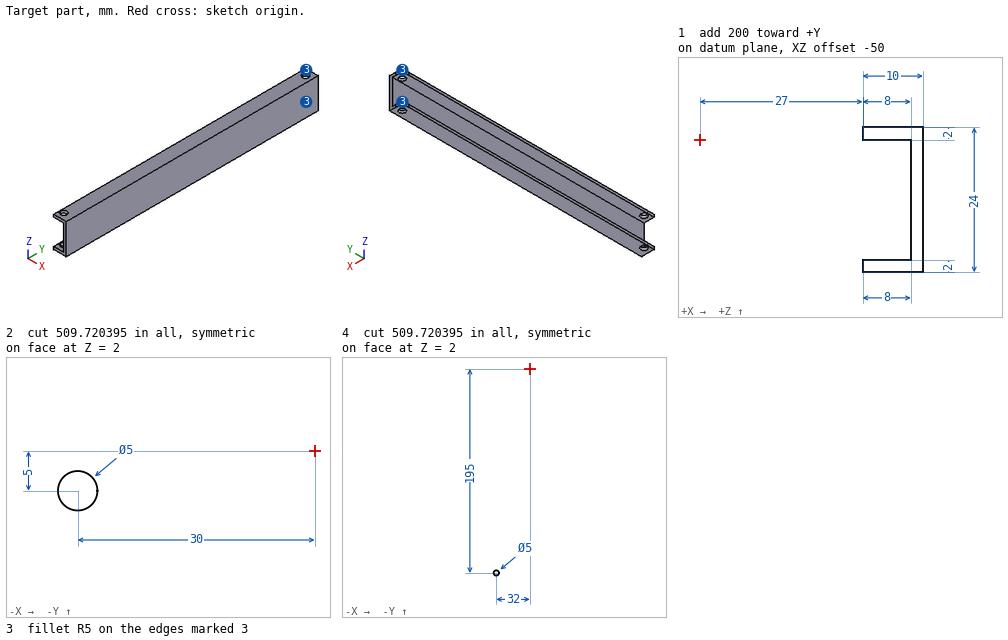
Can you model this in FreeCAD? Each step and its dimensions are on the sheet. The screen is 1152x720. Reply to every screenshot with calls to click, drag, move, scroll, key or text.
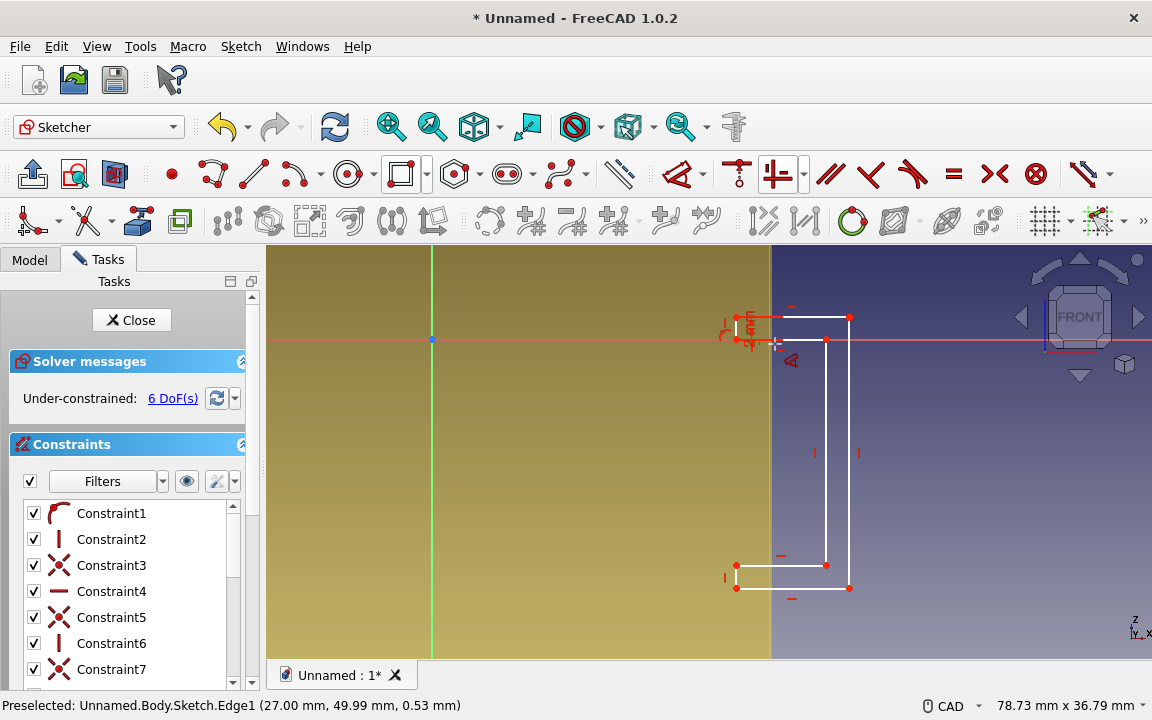
scroll(736, 582, up, 4)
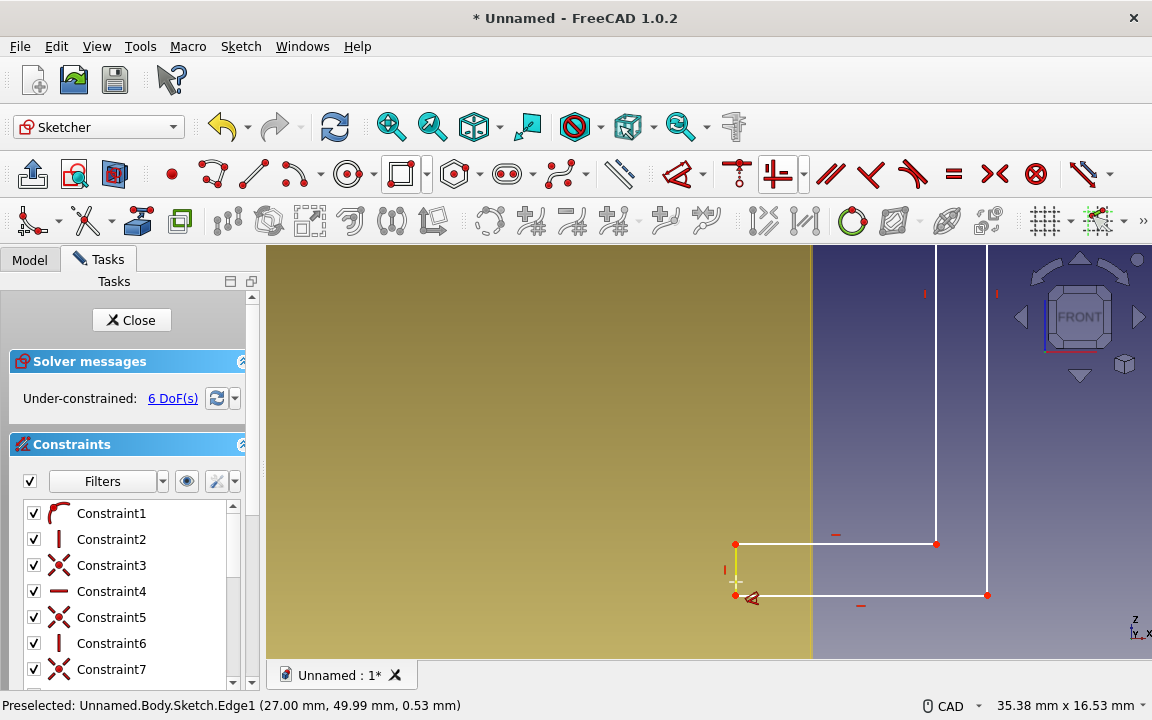
click(736, 580)
click(770, 570)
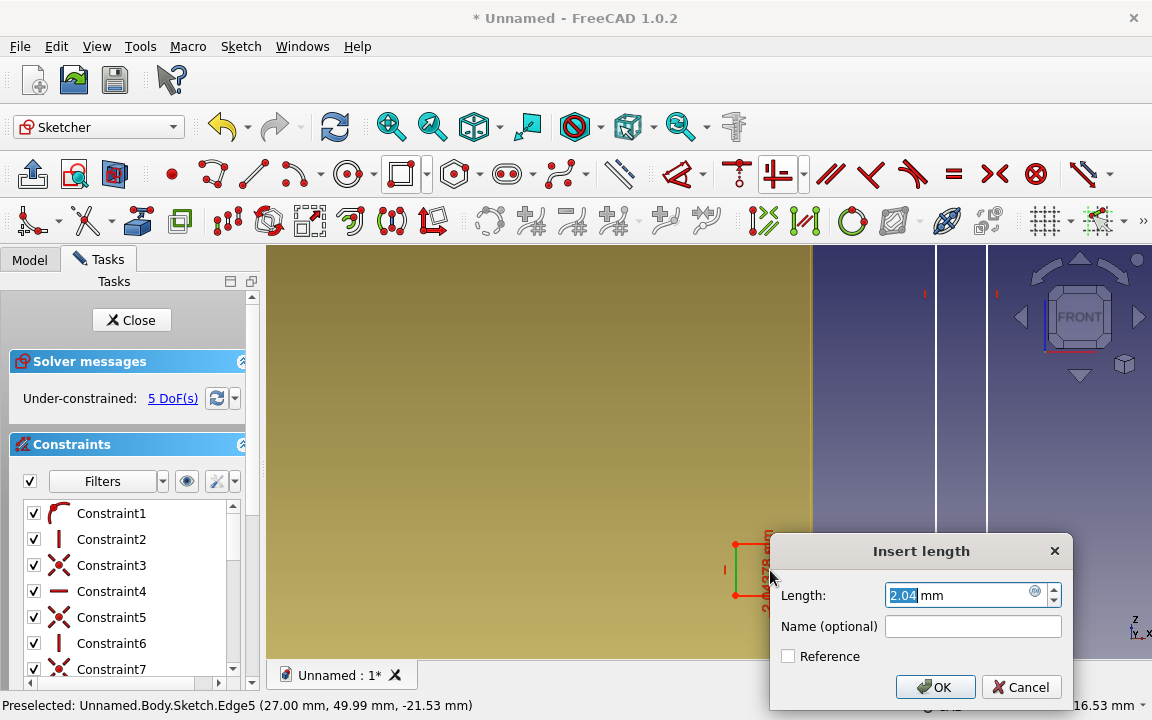
text(2)
key(Return)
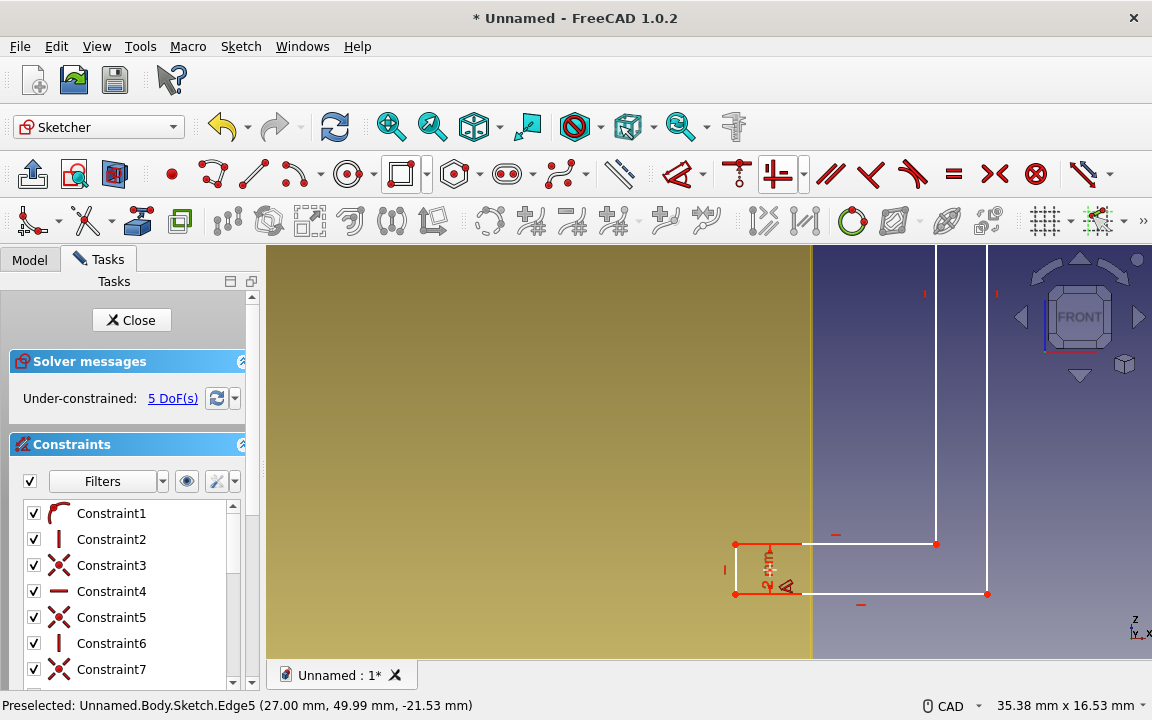
click(796, 544)
click(882, 578)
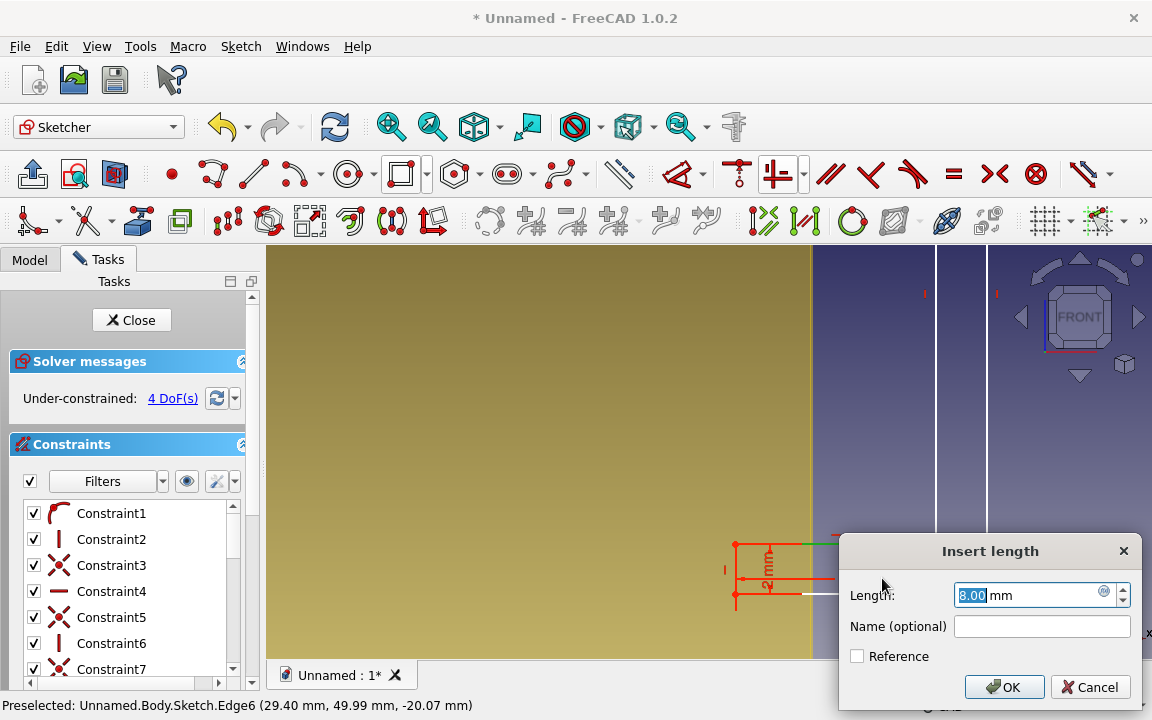
text(8)
key(Return)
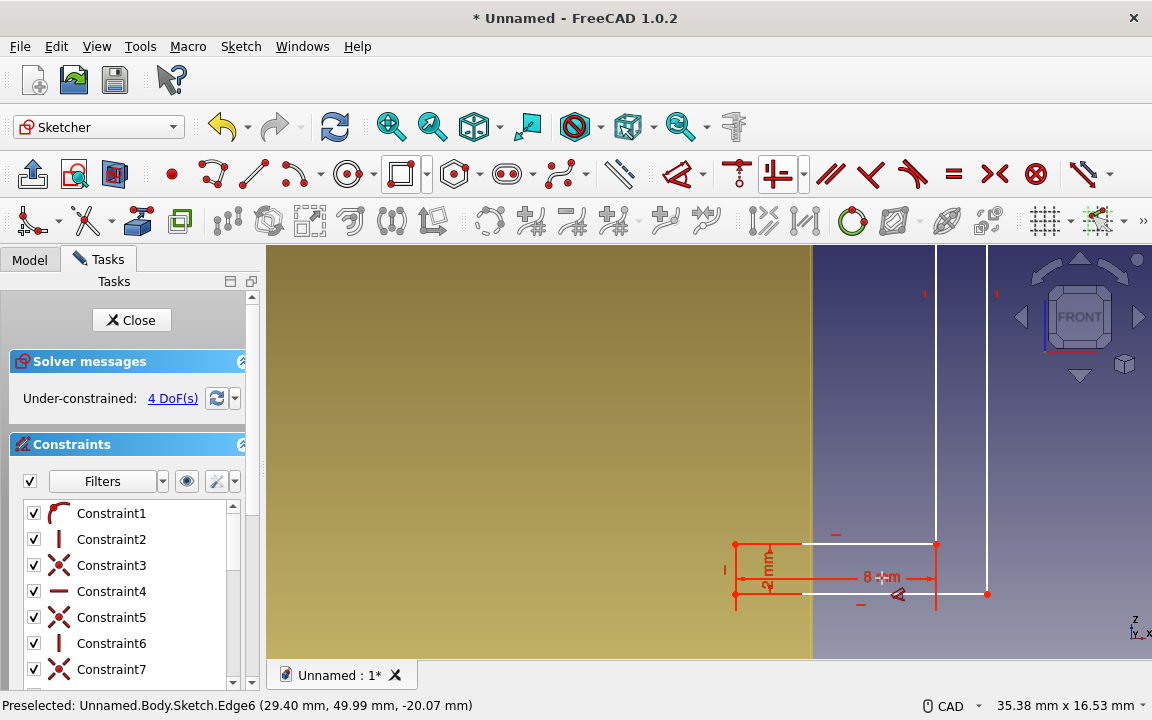
scroll(736, 582, down, 4)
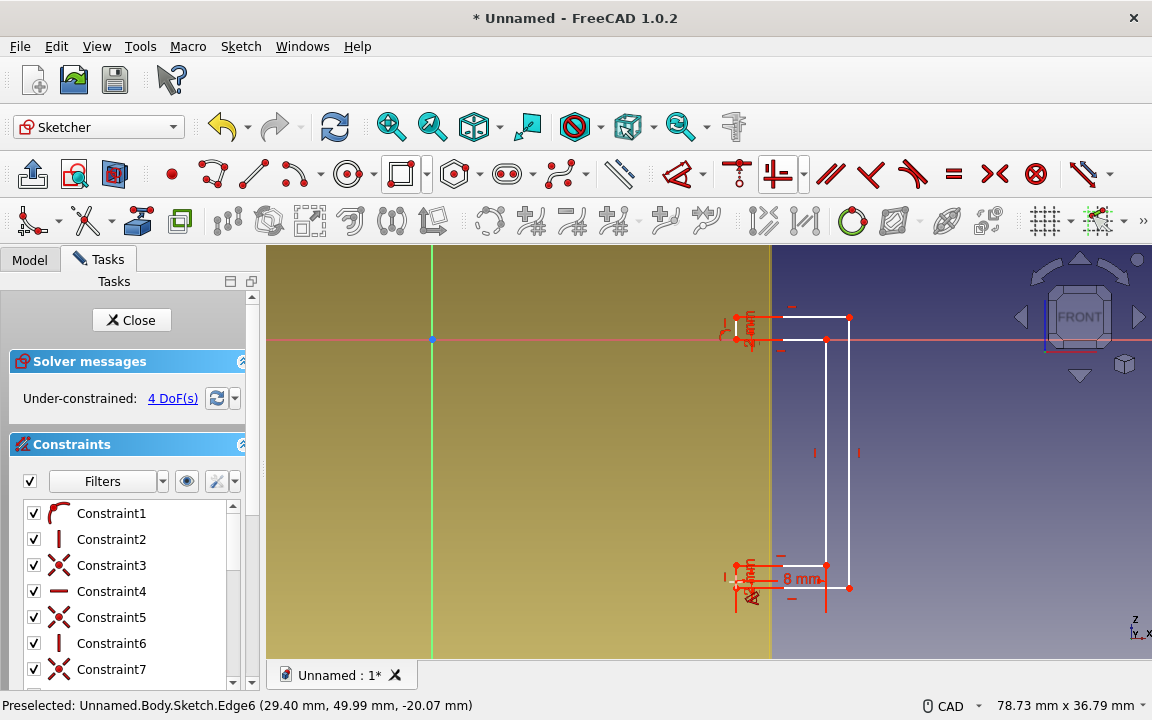
click(799, 340)
click(781, 374)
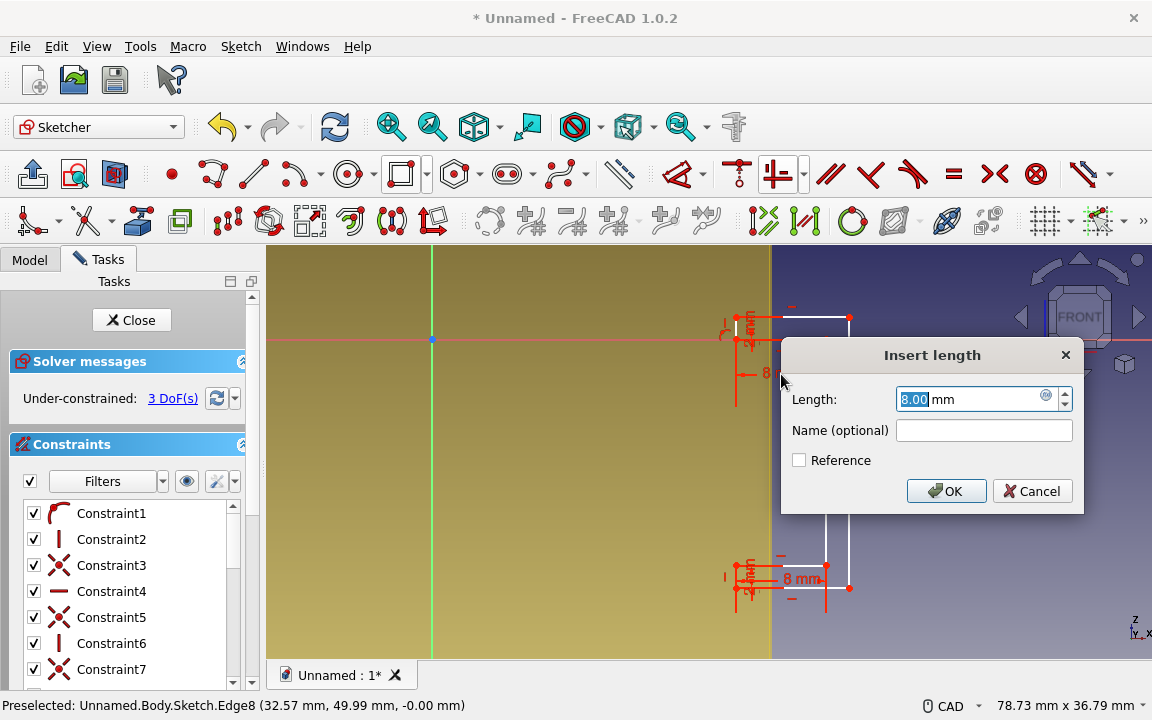
text(8)
key(Return)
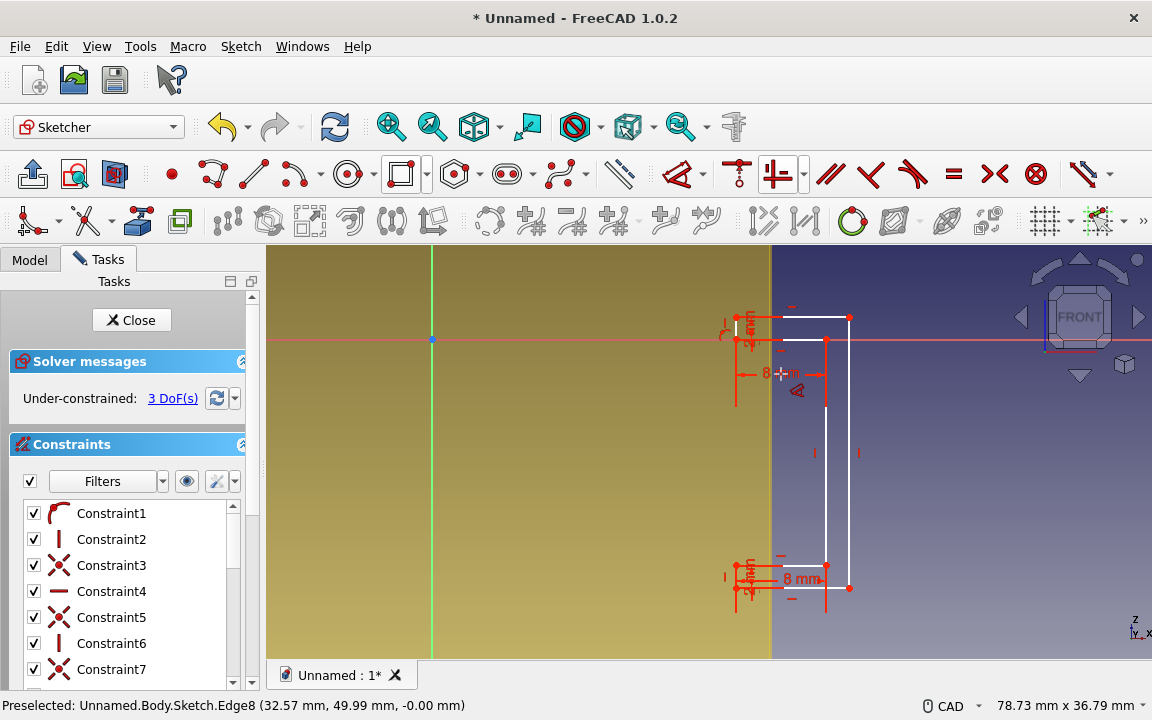
click(770, 317)
click(793, 283)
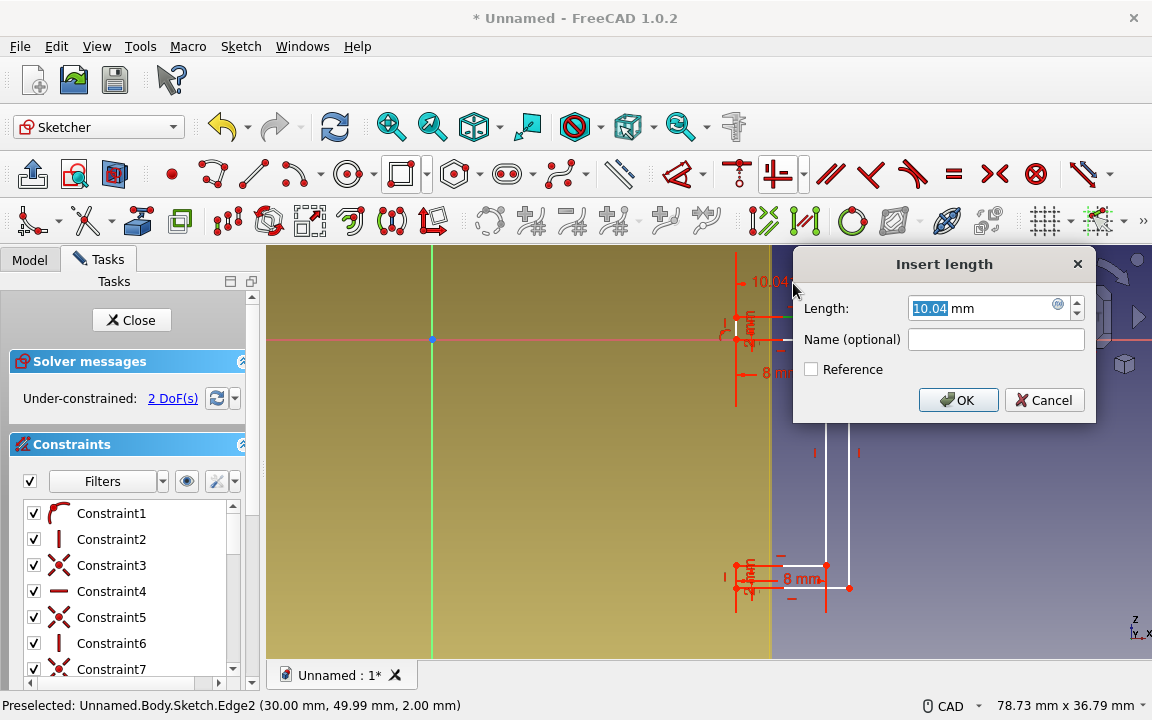
text(10)
key(Return)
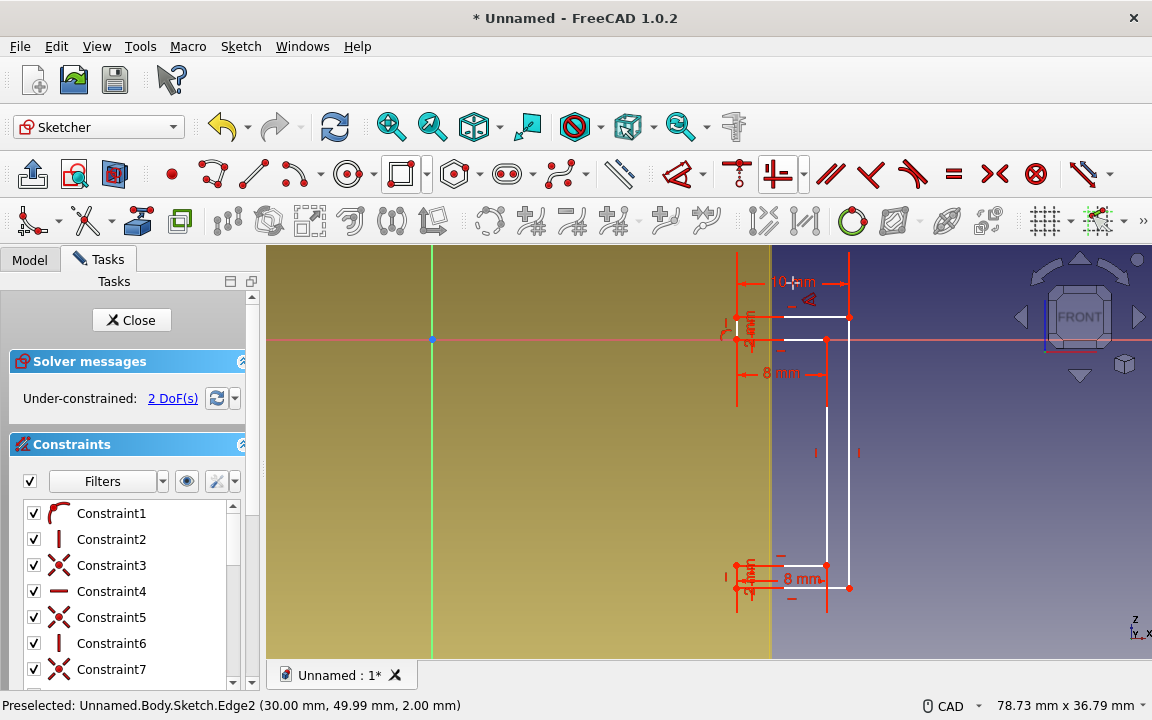
click(849, 398)
click(883, 453)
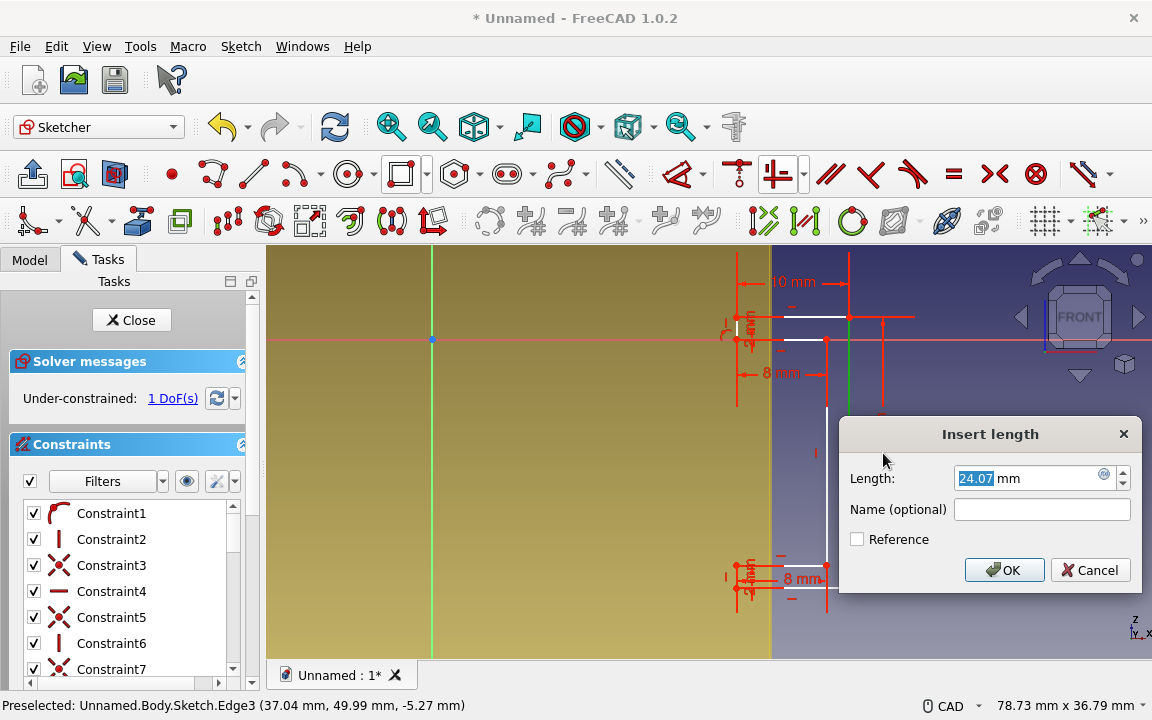
text(24)
key(Return)